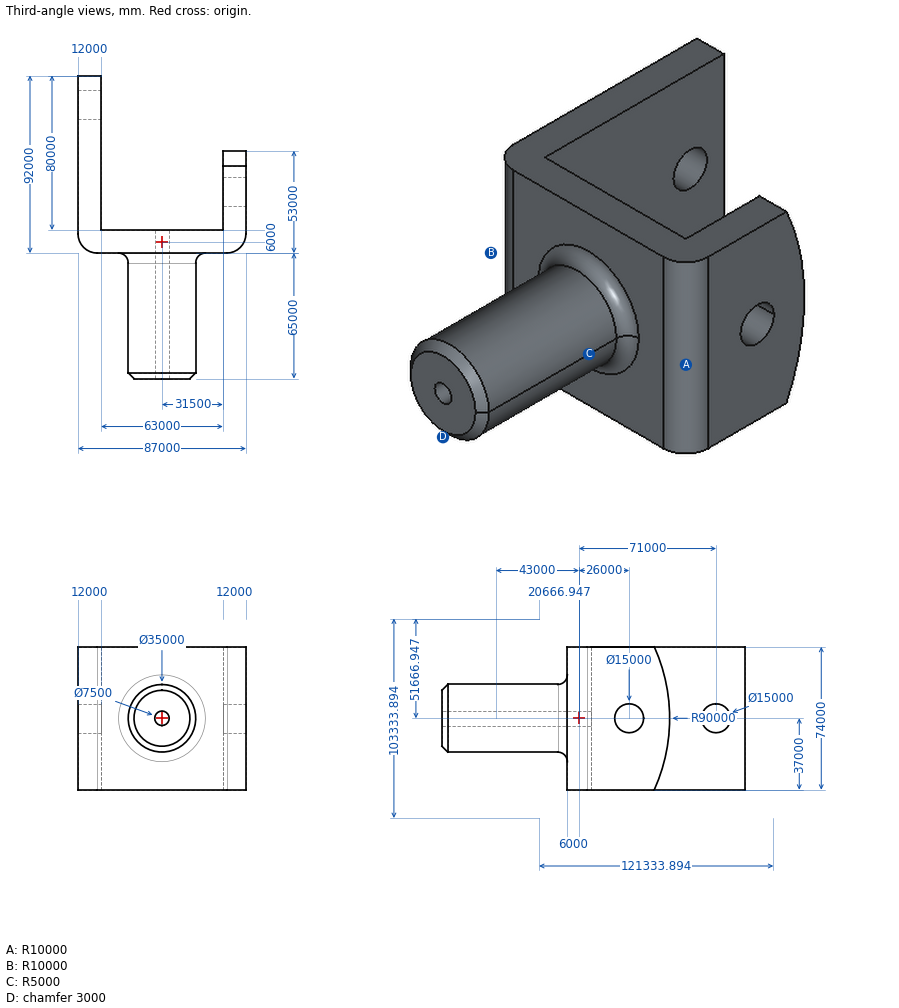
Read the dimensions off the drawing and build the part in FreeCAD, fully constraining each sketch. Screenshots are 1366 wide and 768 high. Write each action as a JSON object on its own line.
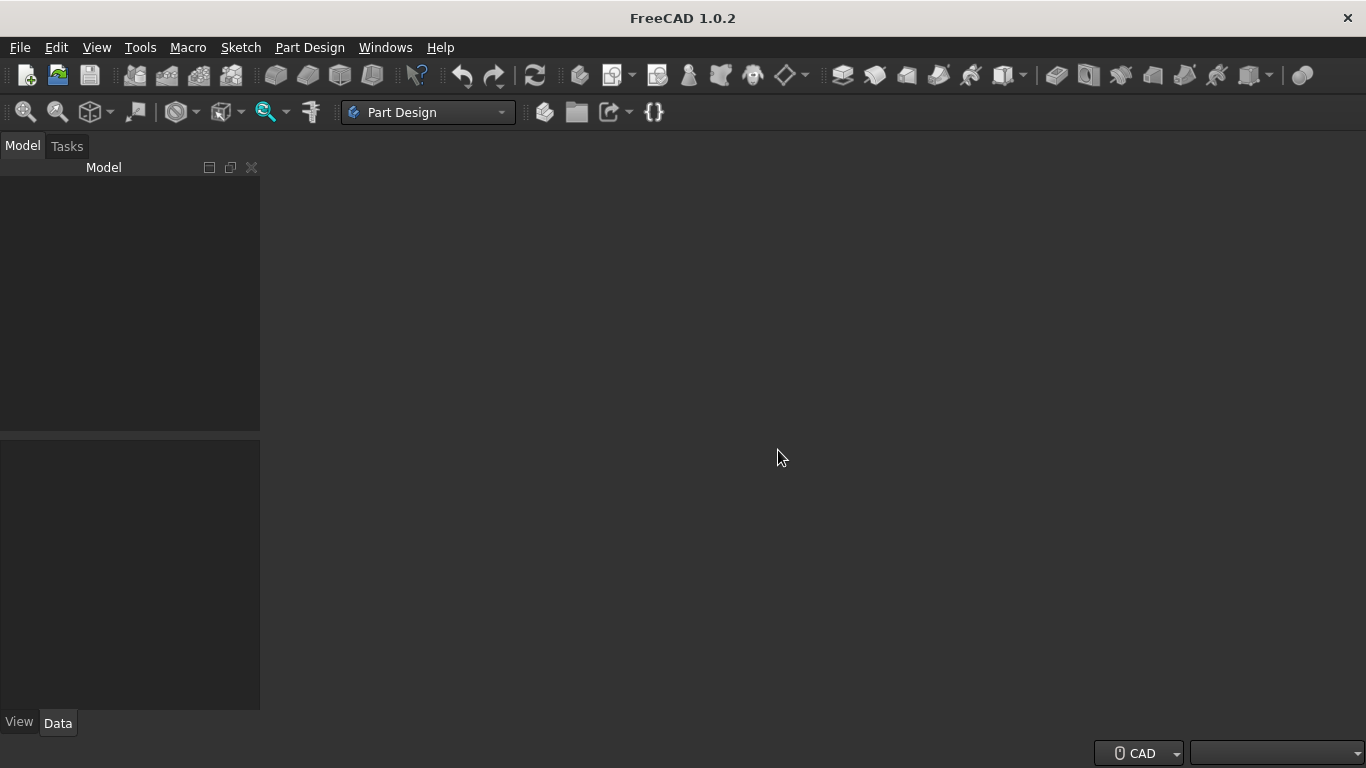
{"action": "left_click", "coordinate": [26, 76]}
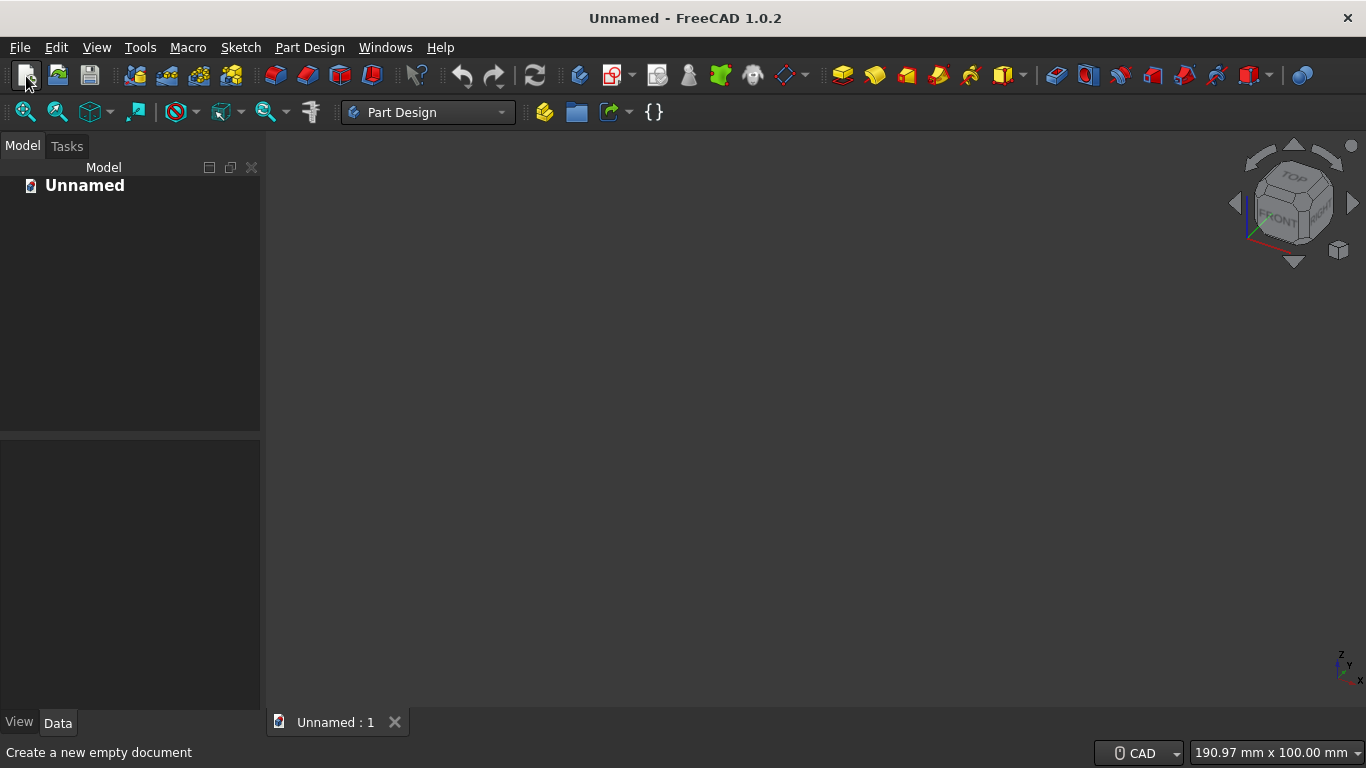
{"action": "left_click", "coordinate": [612, 76]}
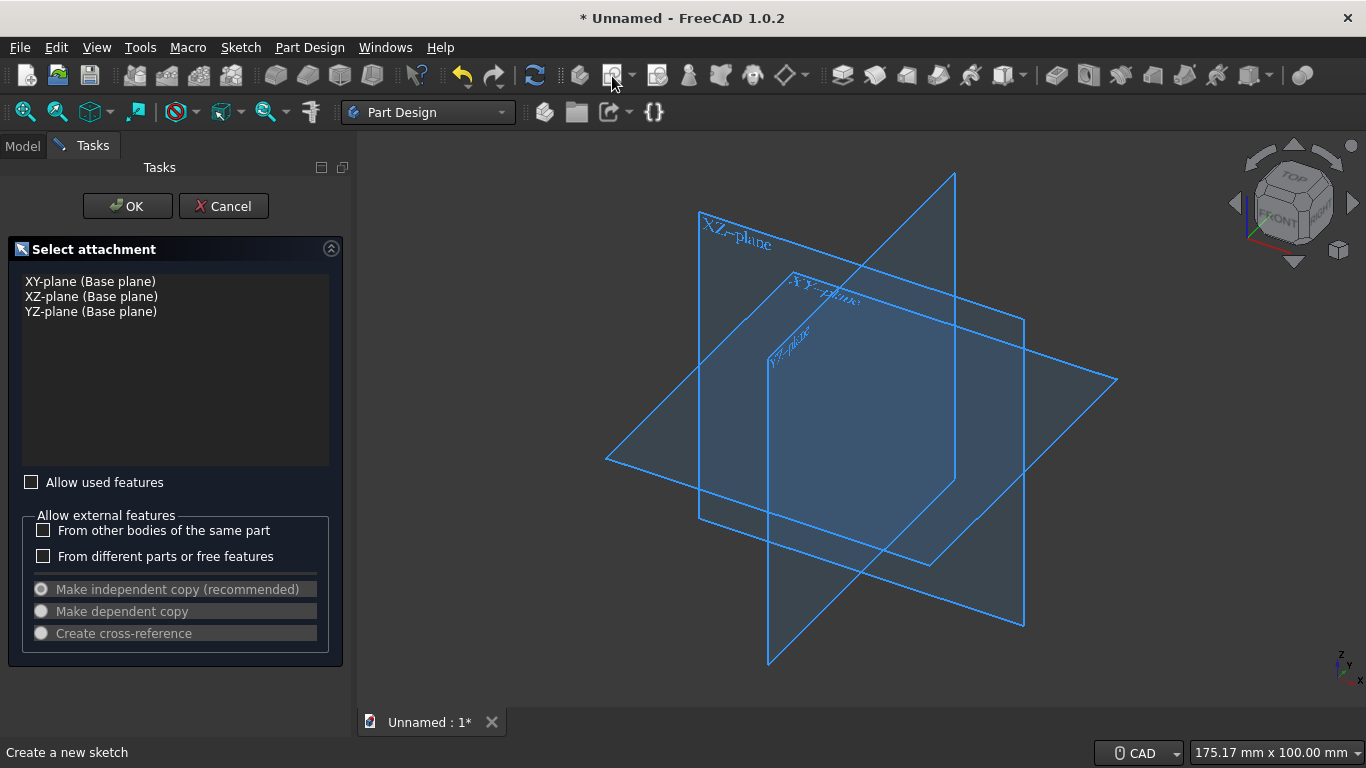
{"action": "left_click", "coordinate": [82, 282]}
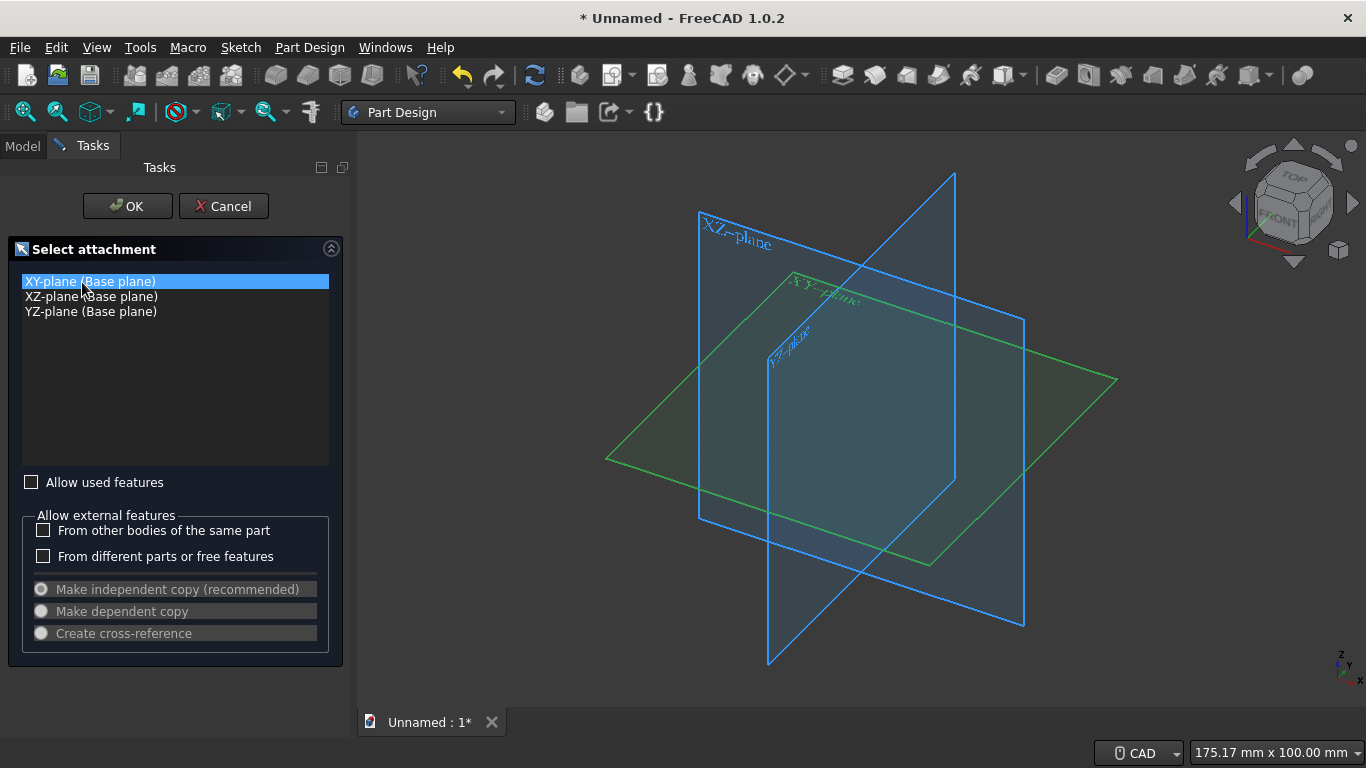
{"action": "left_click", "coordinate": [128, 206]}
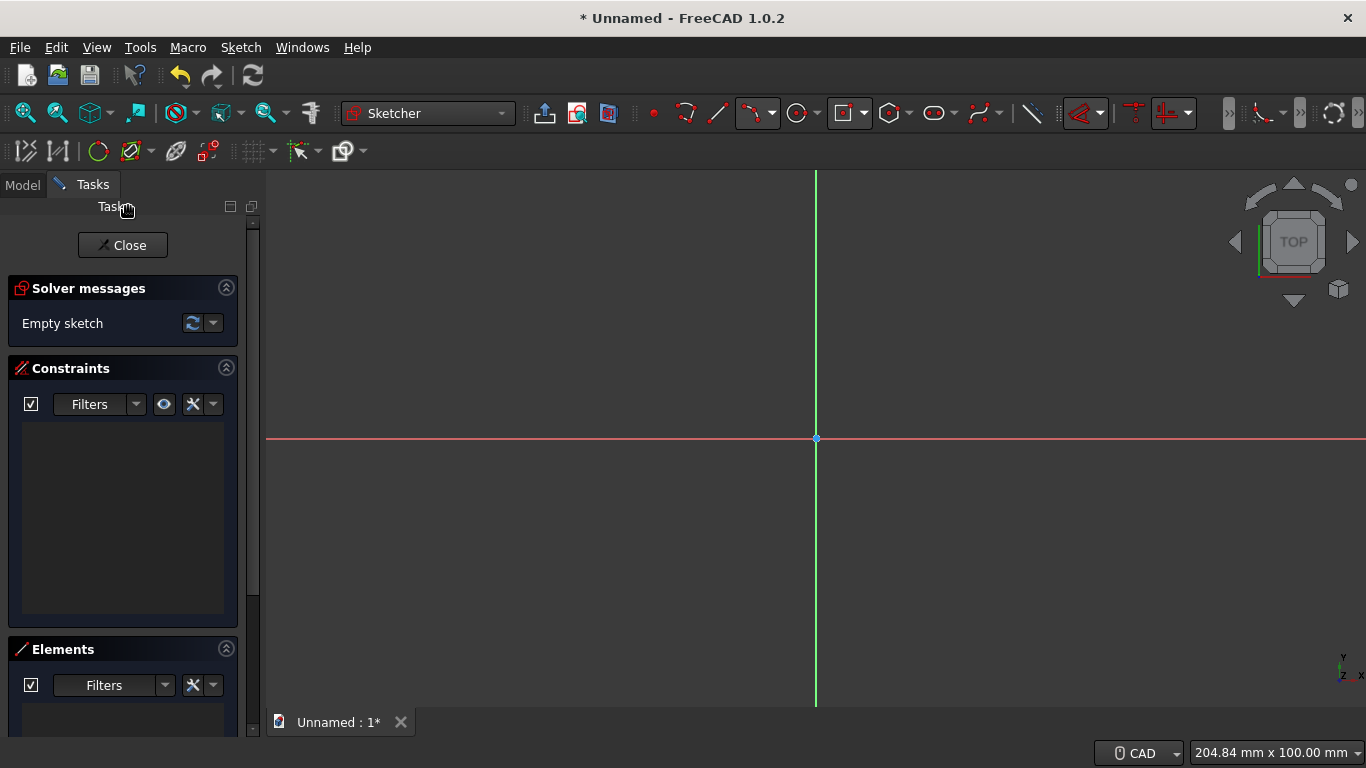
{"action": "scroll", "coordinate": [748, 438], "scroll_direction": "down", "scroll_amount": 15}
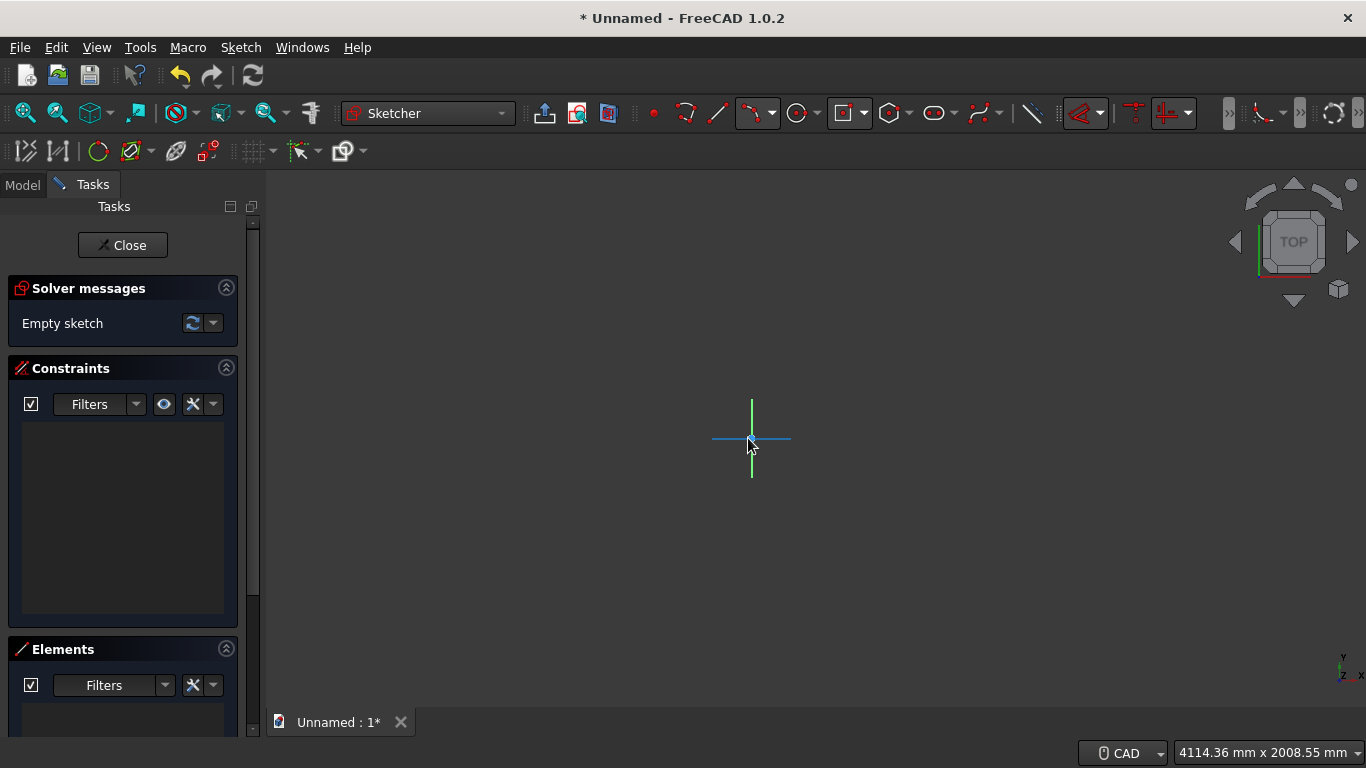
{"action": "scroll", "coordinate": [748, 438], "scroll_direction": "down", "scroll_amount": 15}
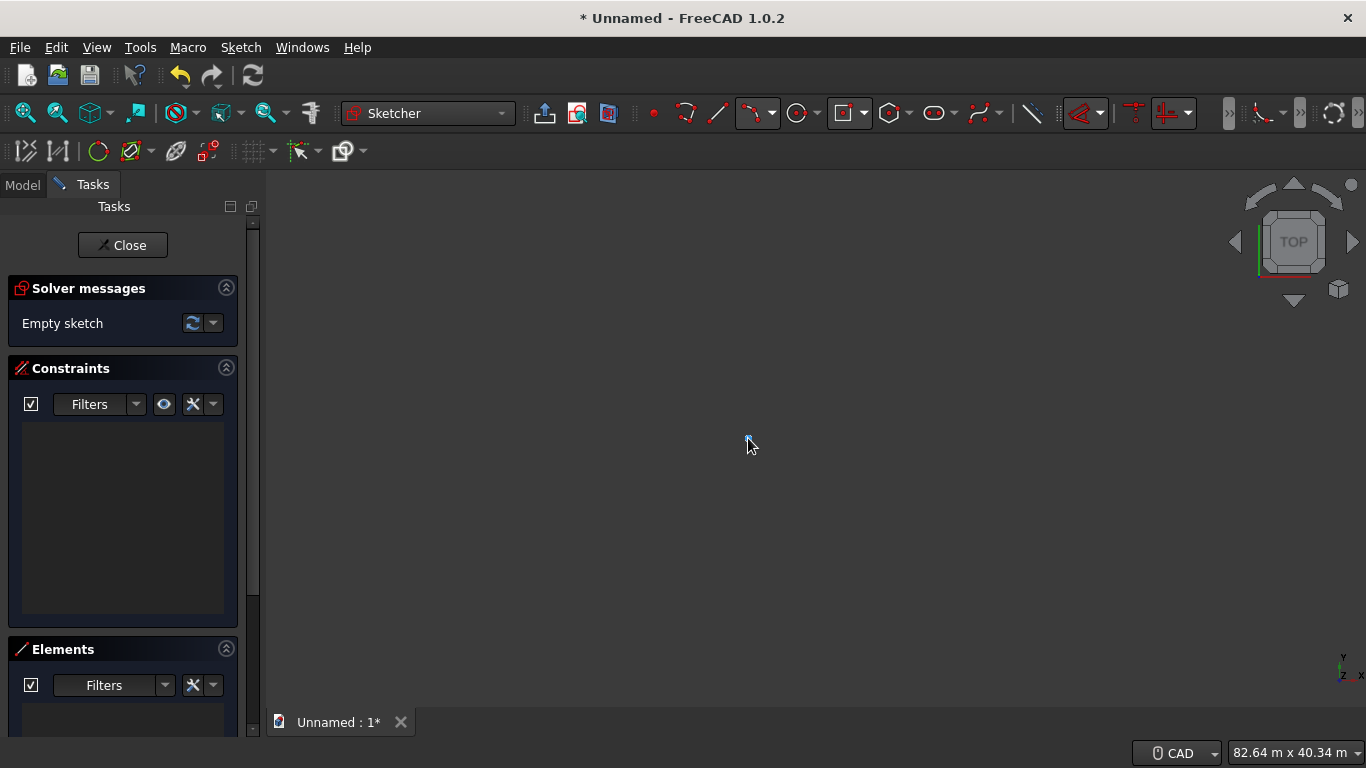
{"action": "scroll", "coordinate": [747, 668], "scroll_direction": "down", "scroll_amount": 6}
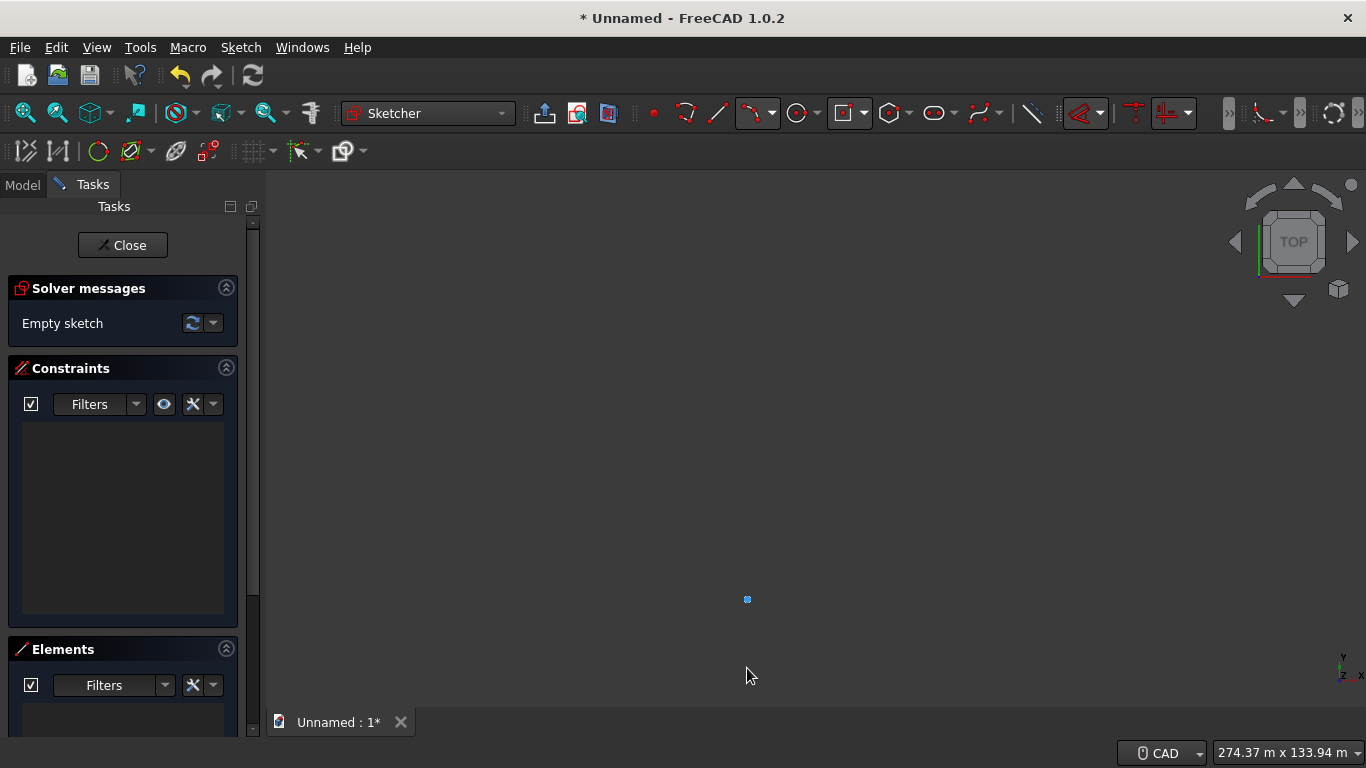
{"action": "left_click", "coordinate": [686, 114]}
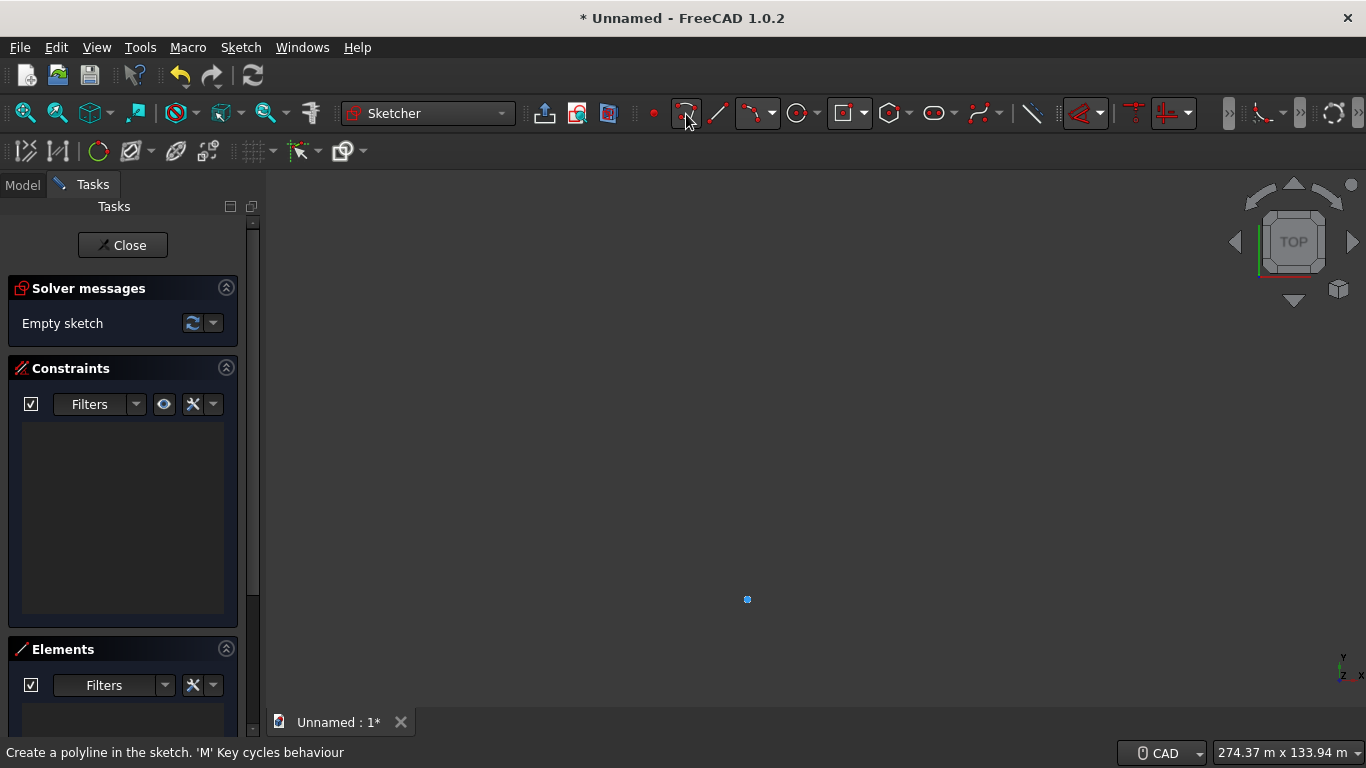
{"action": "left_click", "coordinate": [874, 575]}
{"action": "left_click", "coordinate": [622, 575]}
{"action": "left_click", "coordinate": [622, 255]}
{"action": "left_click", "coordinate": [573, 255]}
{"action": "left_click", "coordinate": [573, 624]}
{"action": "left_click", "coordinate": [922, 624]}
{"action": "left_click", "coordinate": [922, 411]}
{"action": "left_click", "coordinate": [874, 411]}
{"action": "left_click", "coordinate": [874, 576]}
{"action": "key", "text": "Escape"}
{"action": "key", "text": "Escape"}